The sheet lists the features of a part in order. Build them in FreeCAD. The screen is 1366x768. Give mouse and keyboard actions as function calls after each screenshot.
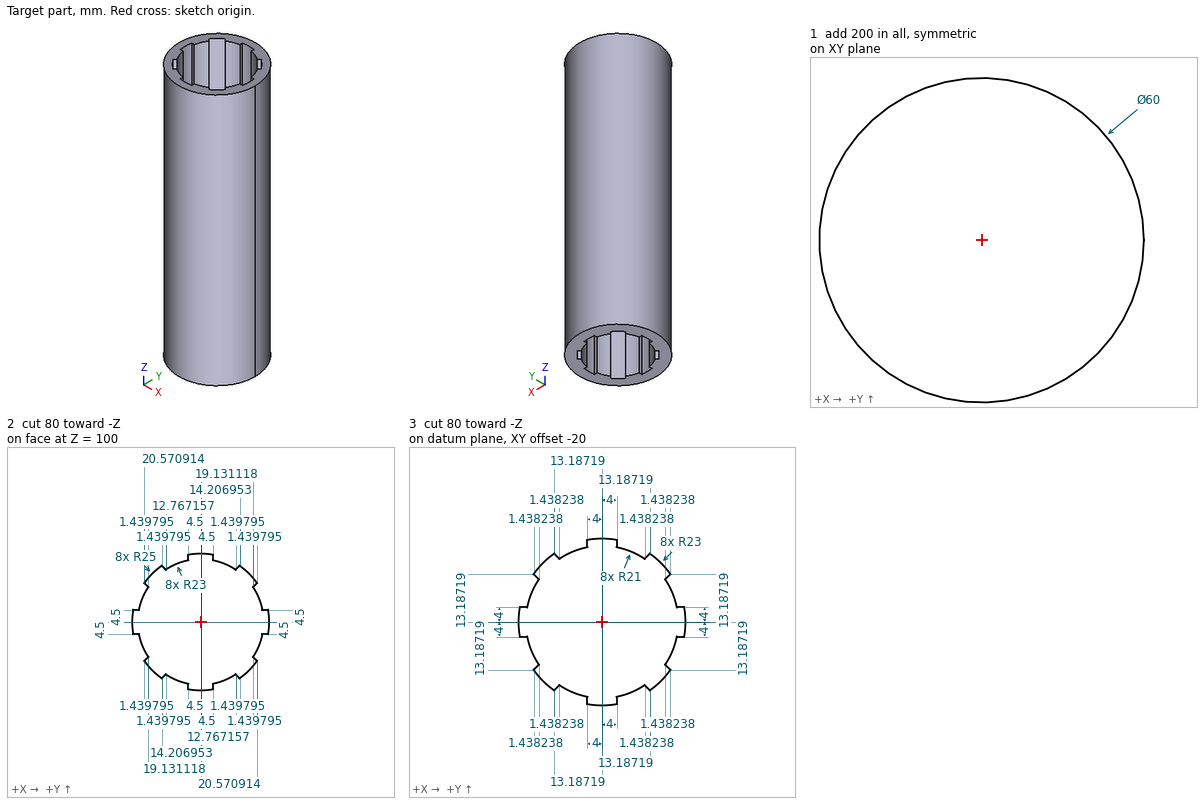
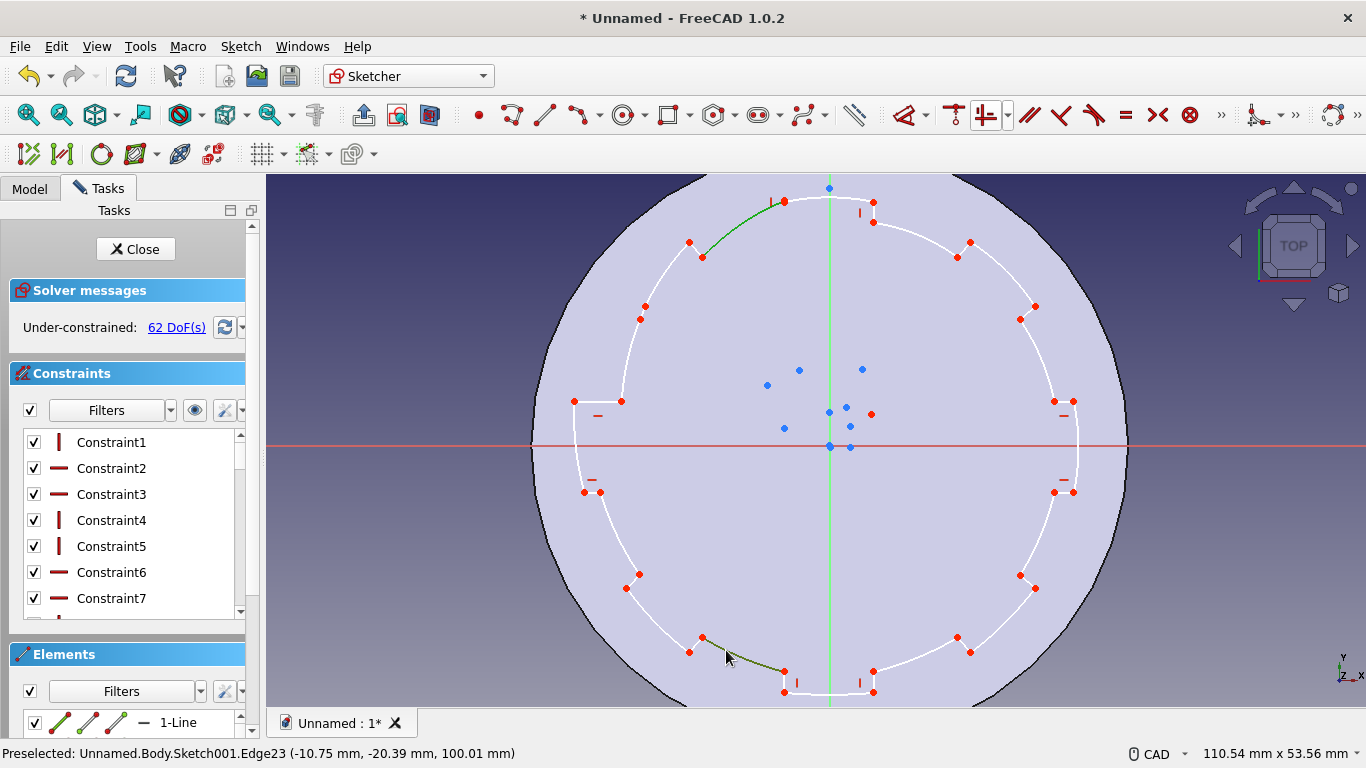
click(954, 116)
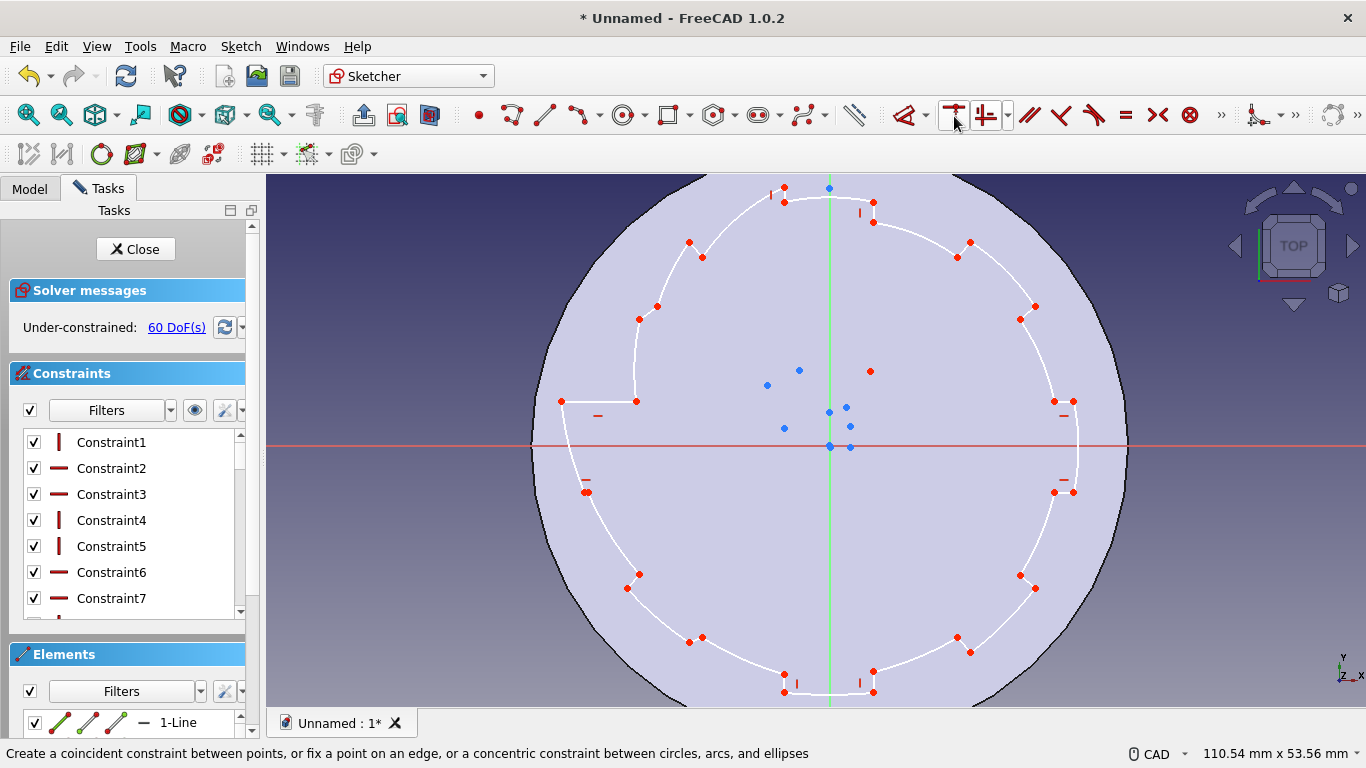
click(756, 203)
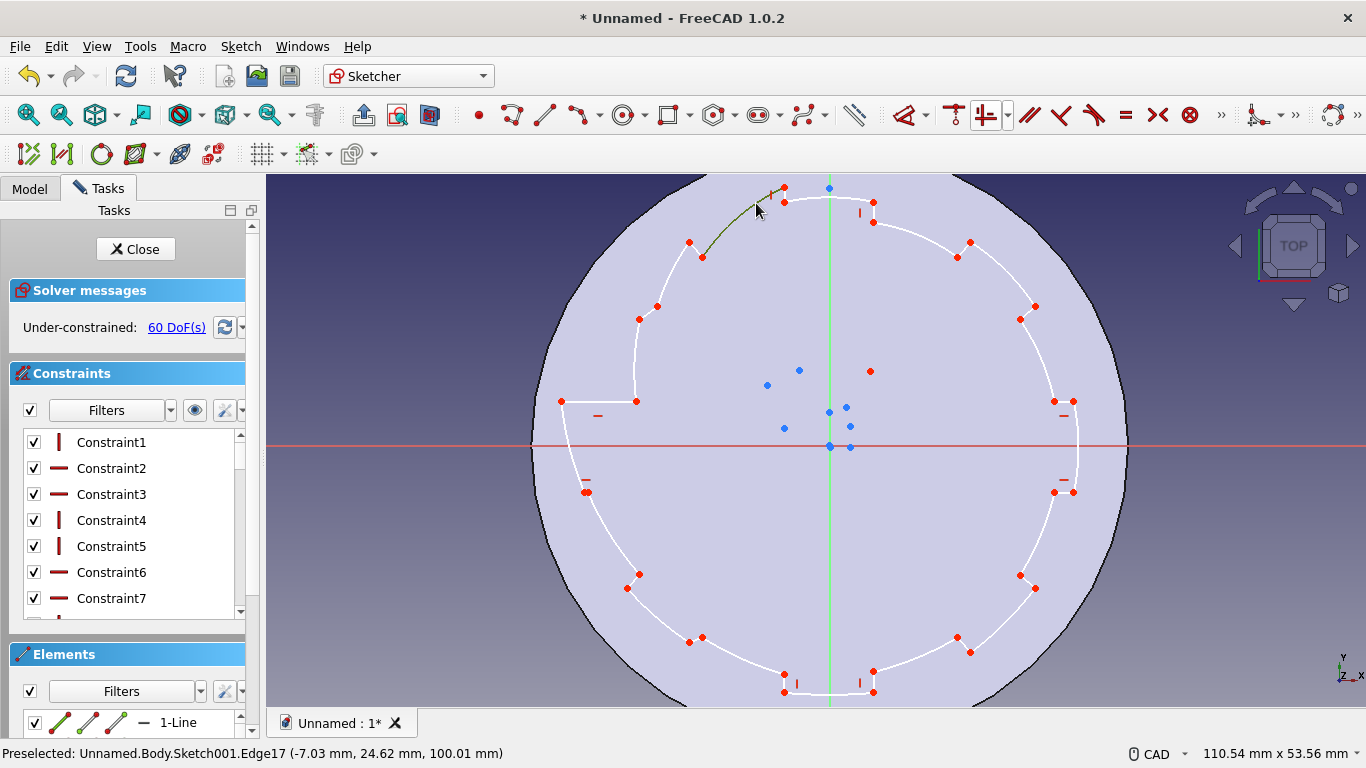
scroll(580, 429, down, 2)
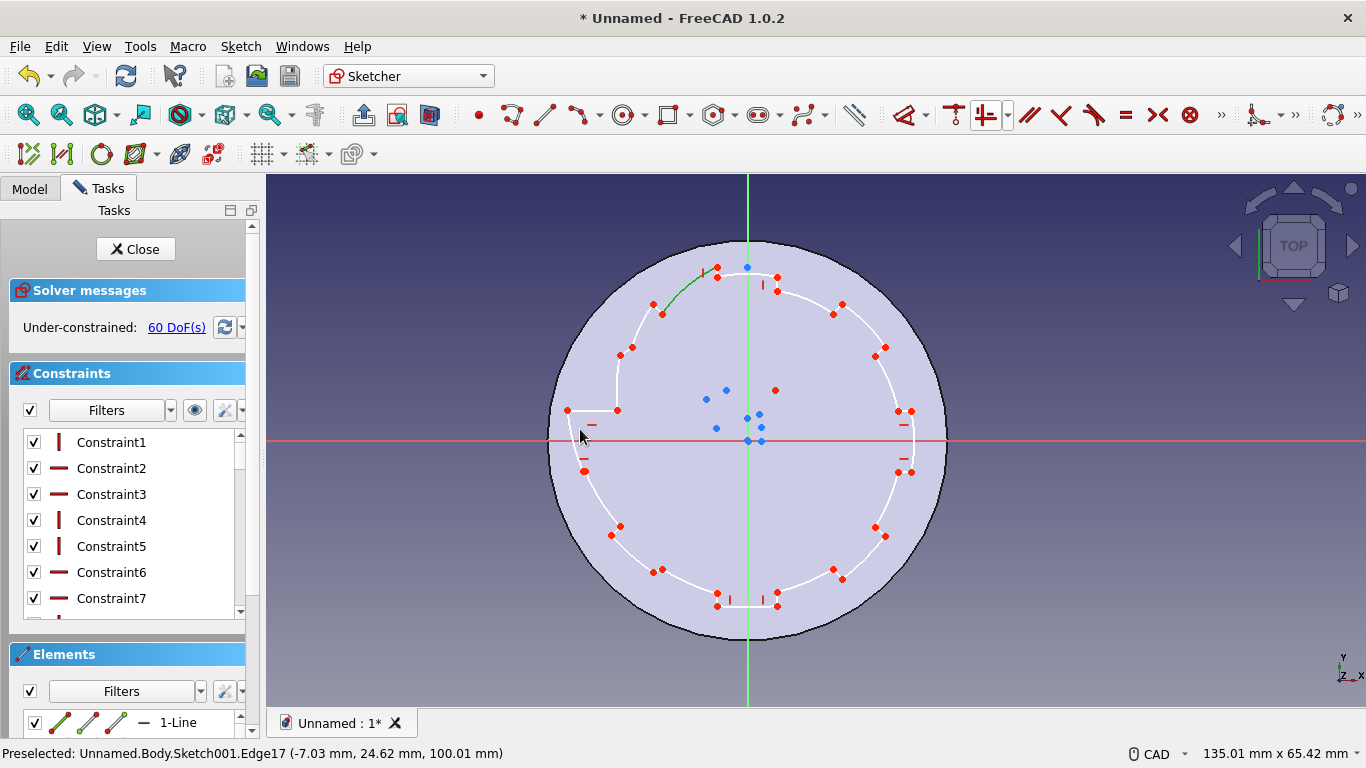
click(735, 607)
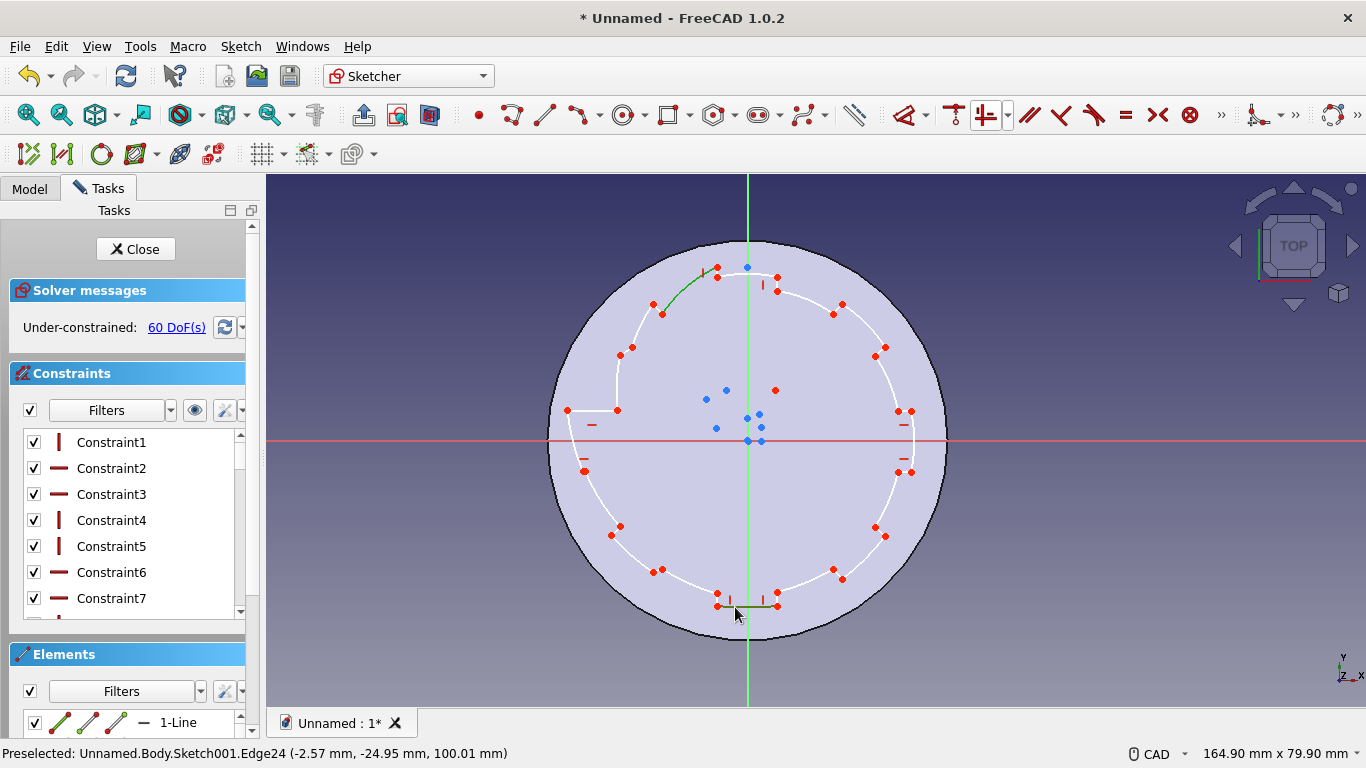
click(954, 116)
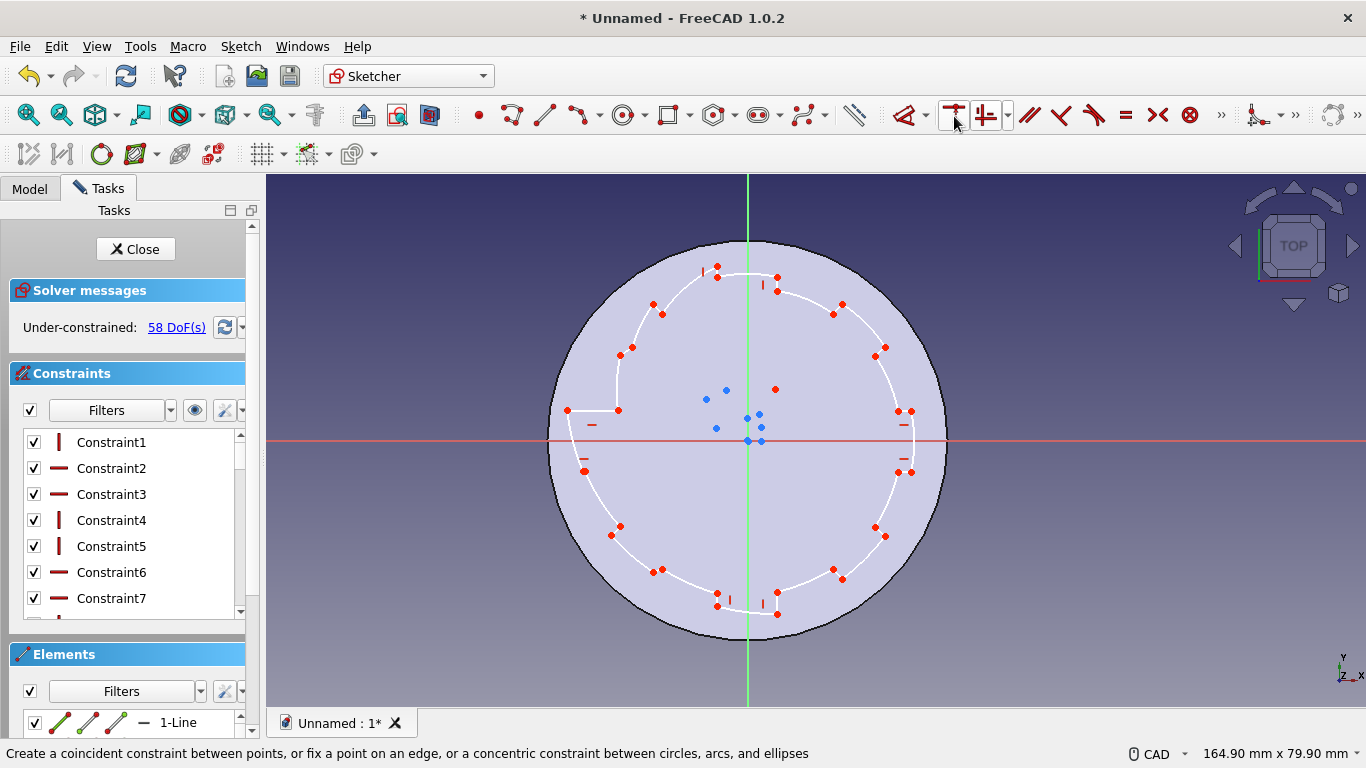
click(698, 278)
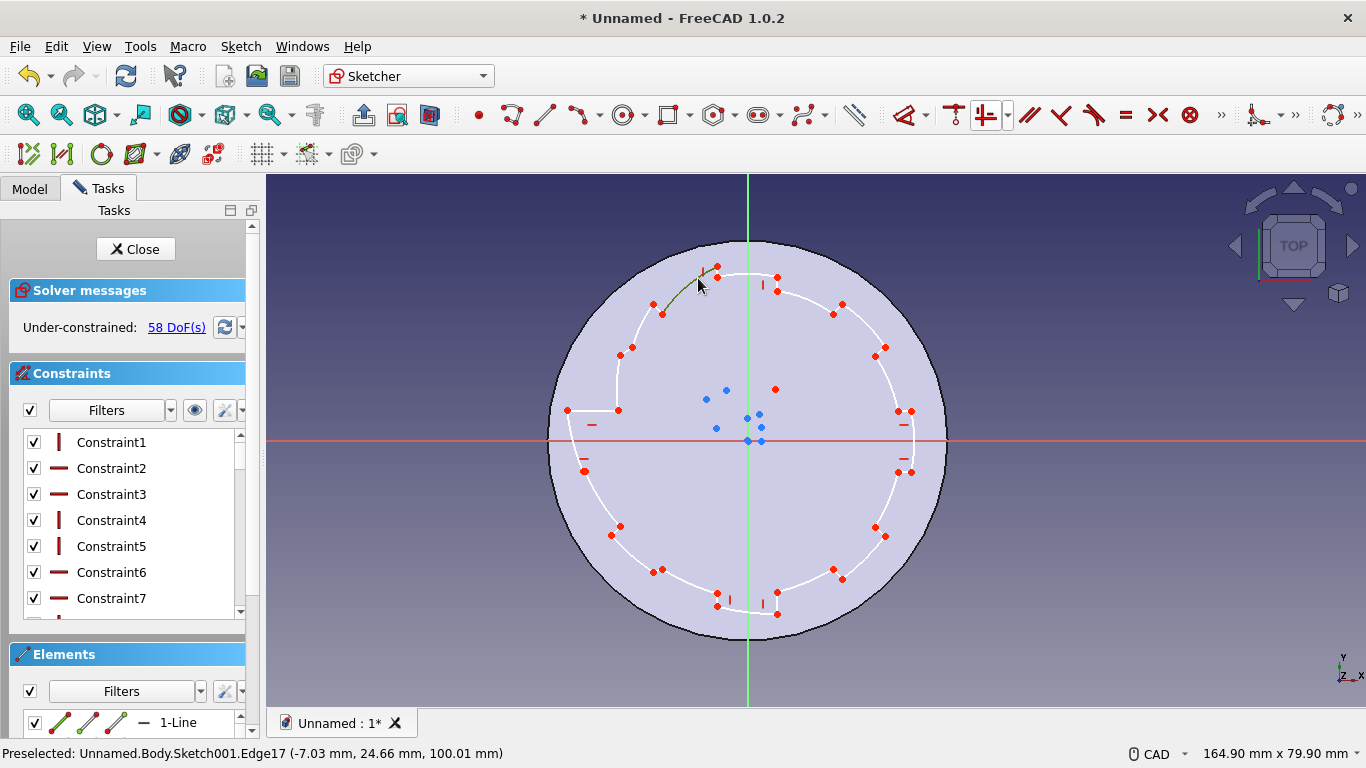
click(795, 587)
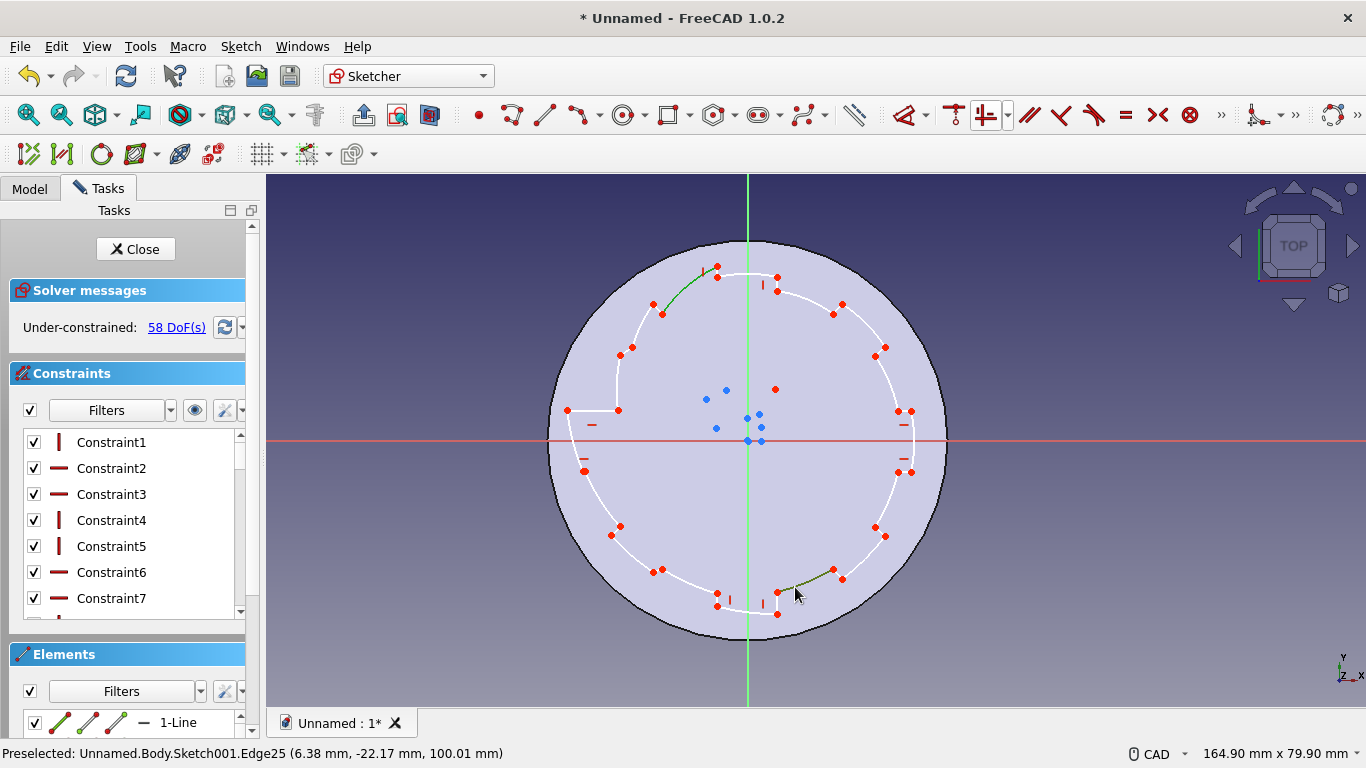
click(954, 116)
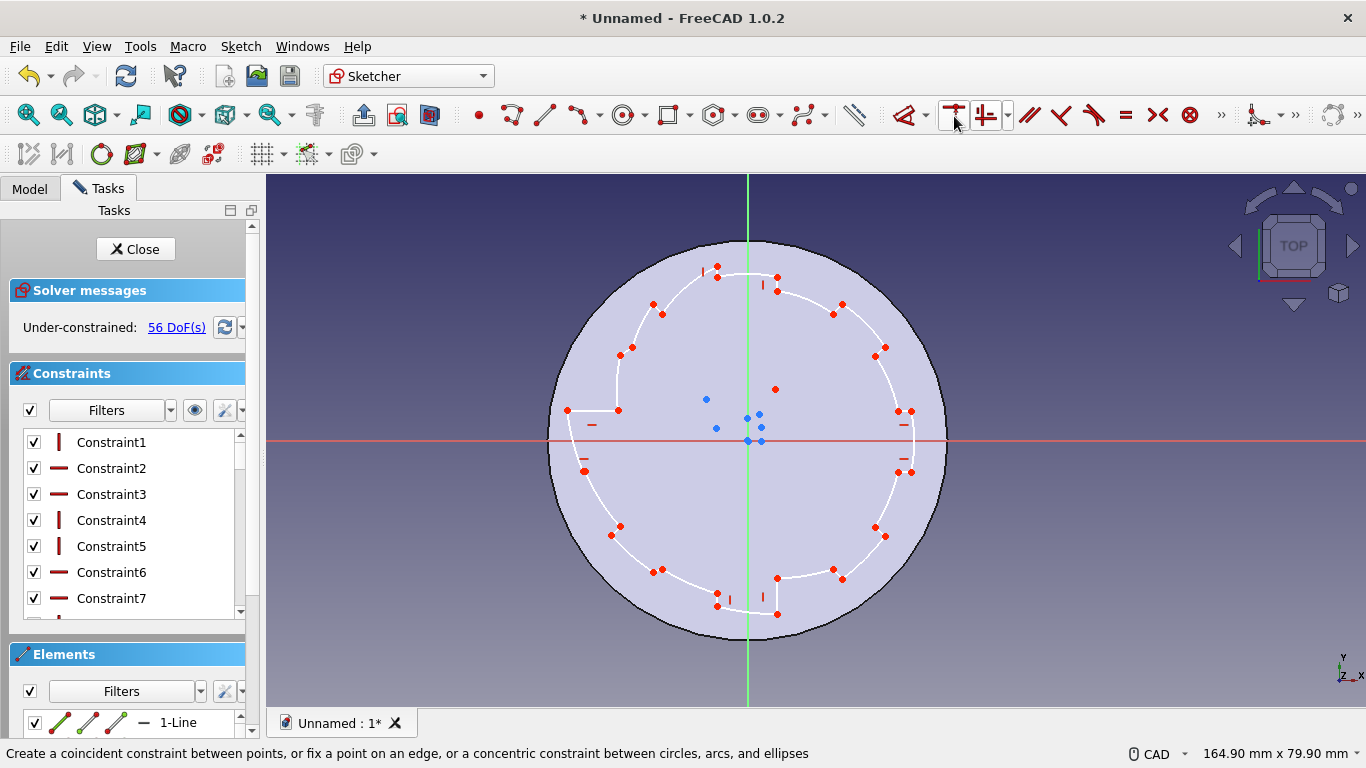
click(698, 278)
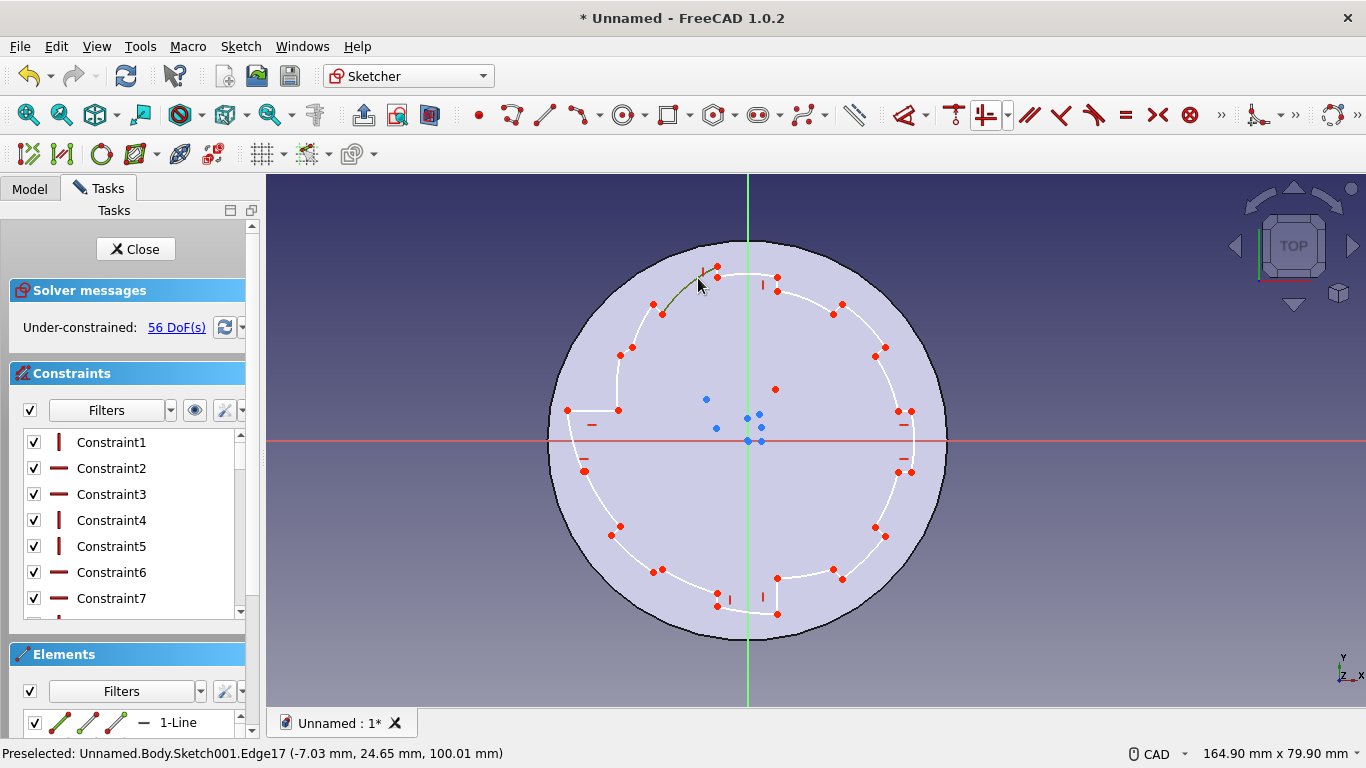
click(856, 567)